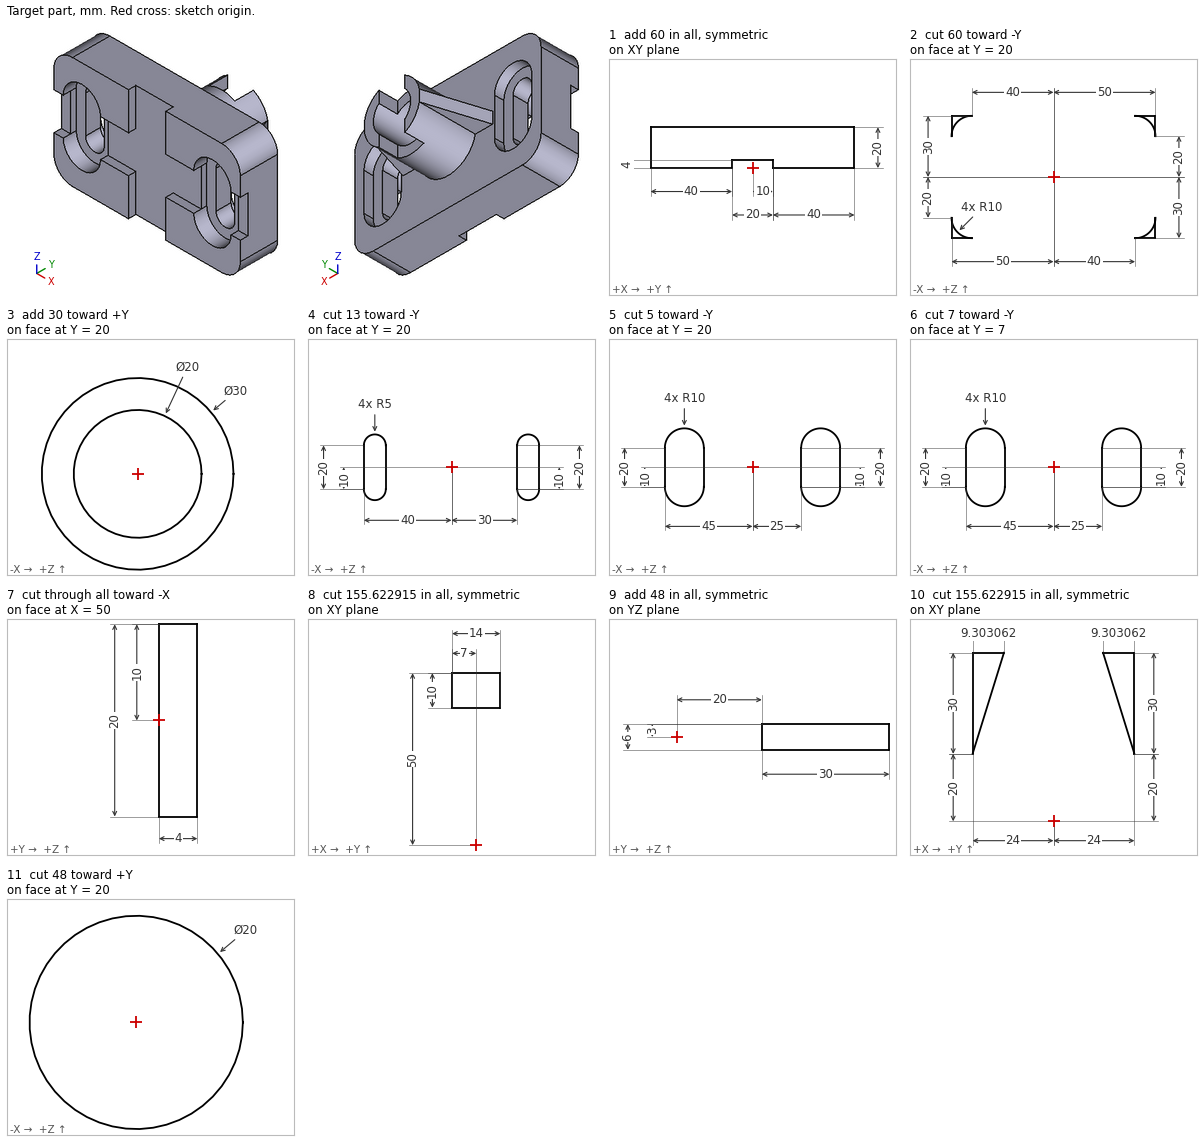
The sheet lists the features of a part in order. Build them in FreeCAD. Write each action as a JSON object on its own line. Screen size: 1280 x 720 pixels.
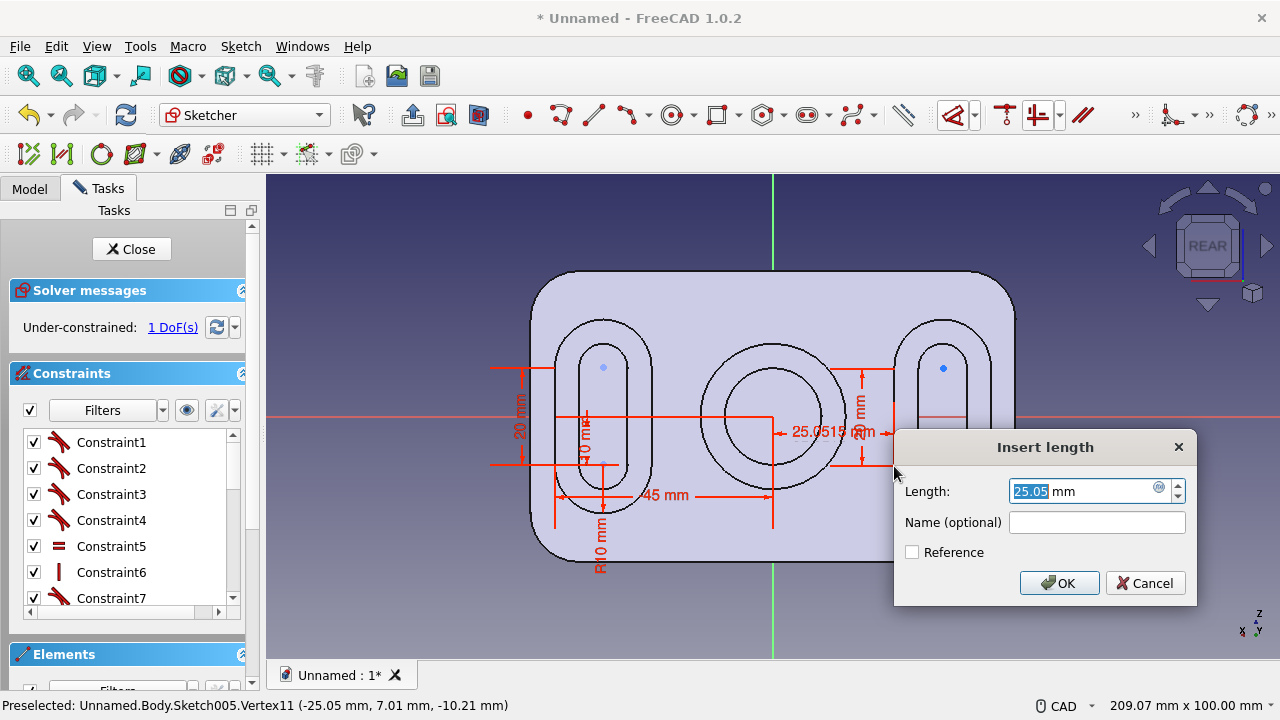
{"action": "type", "text": "25"}
{"action": "key", "text": "Return"}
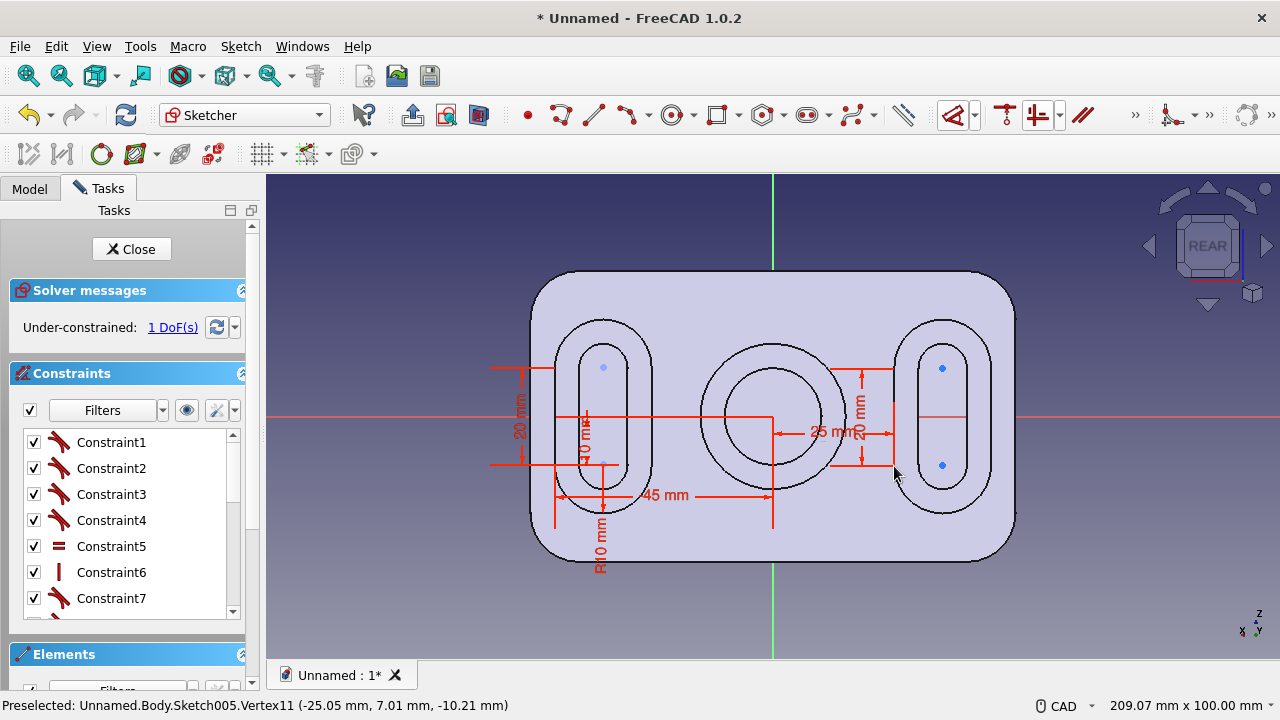
{"action": "left_click", "coordinate": [894, 466]}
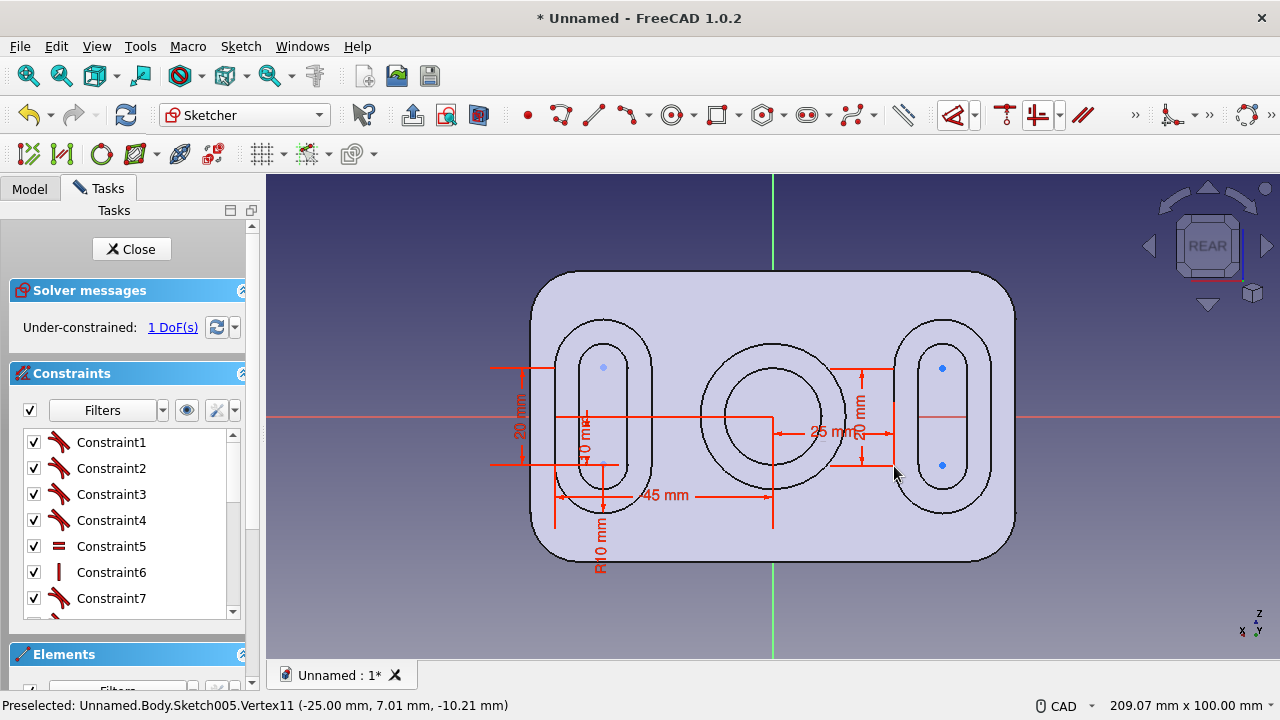
{"action": "key", "text": "i"}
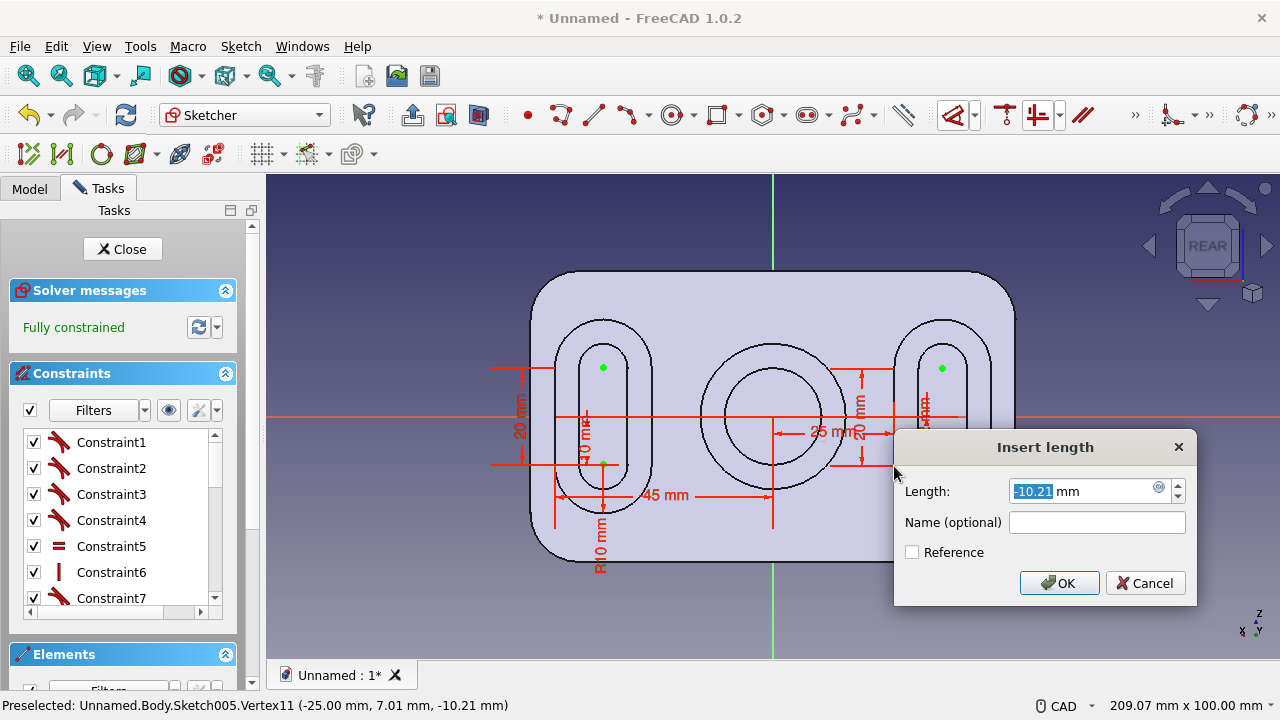
{"action": "type", "text": "-10"}
{"action": "key", "text": "Return"}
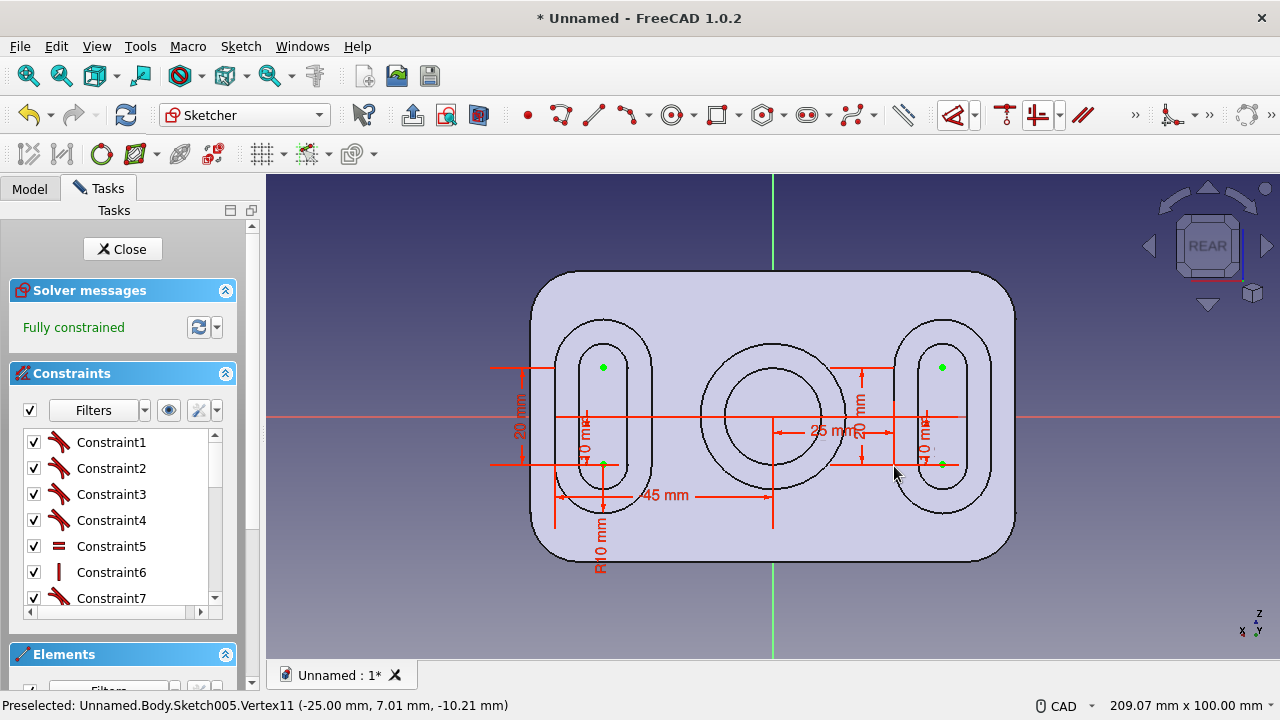
{"action": "left_click", "coordinate": [123, 249]}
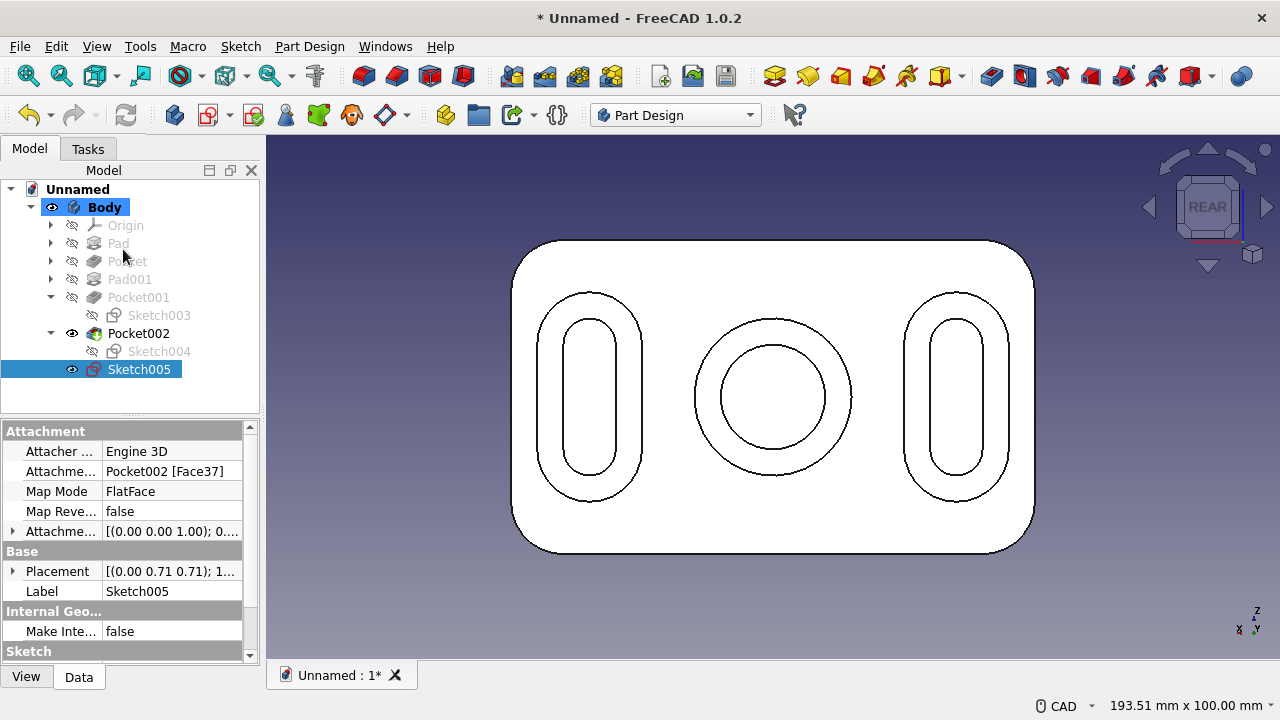
{"action": "left_click", "coordinate": [992, 76]}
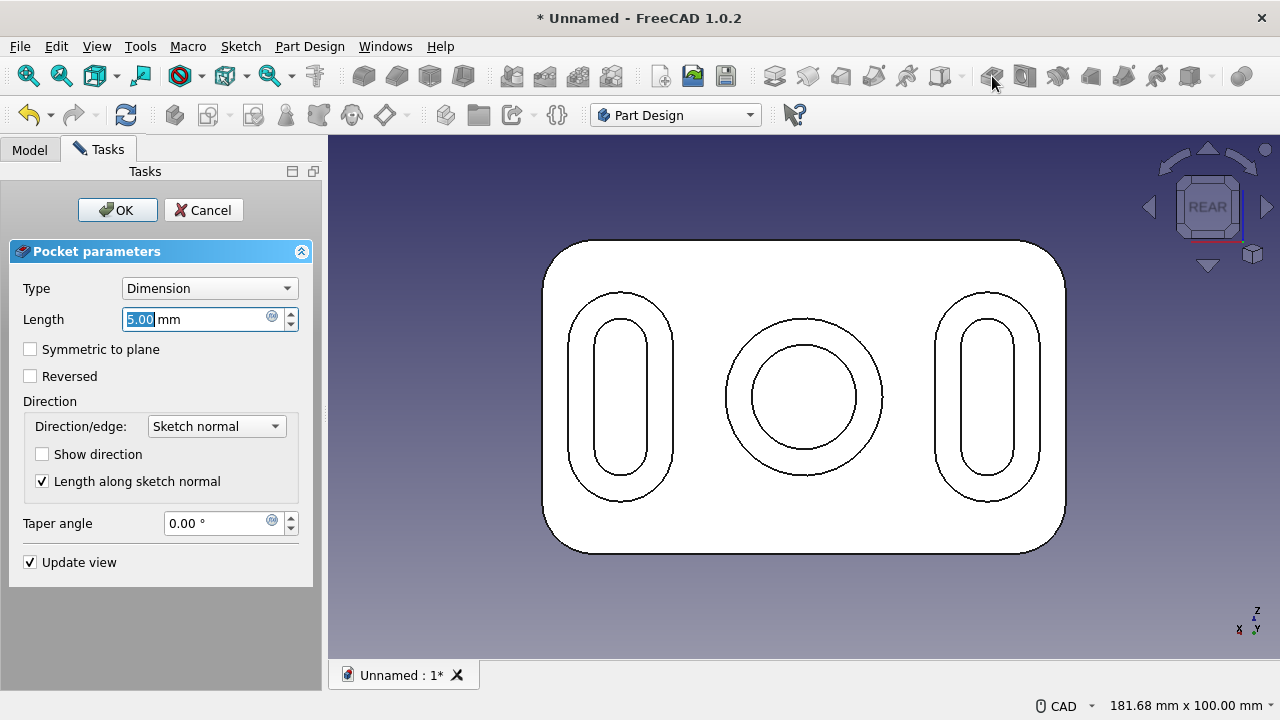
{"action": "type", "text": "7"}
{"action": "key", "text": "Tab"}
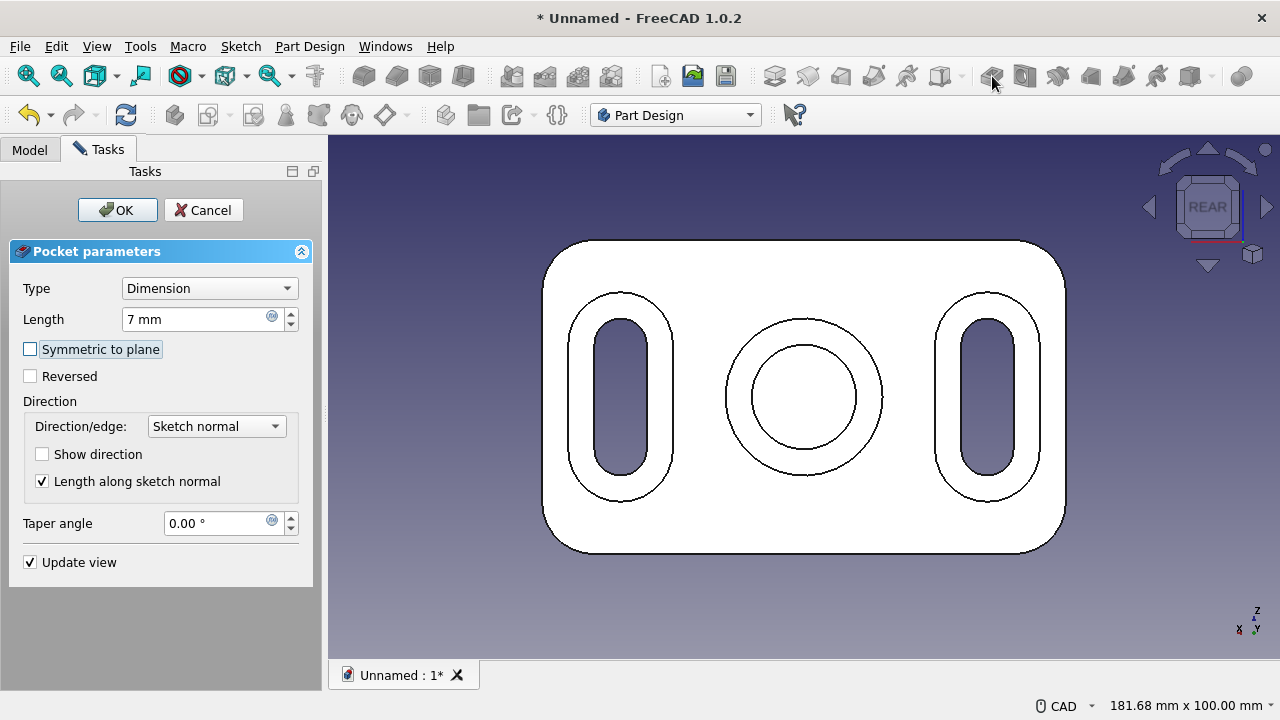
{"action": "left_click", "coordinate": [118, 210]}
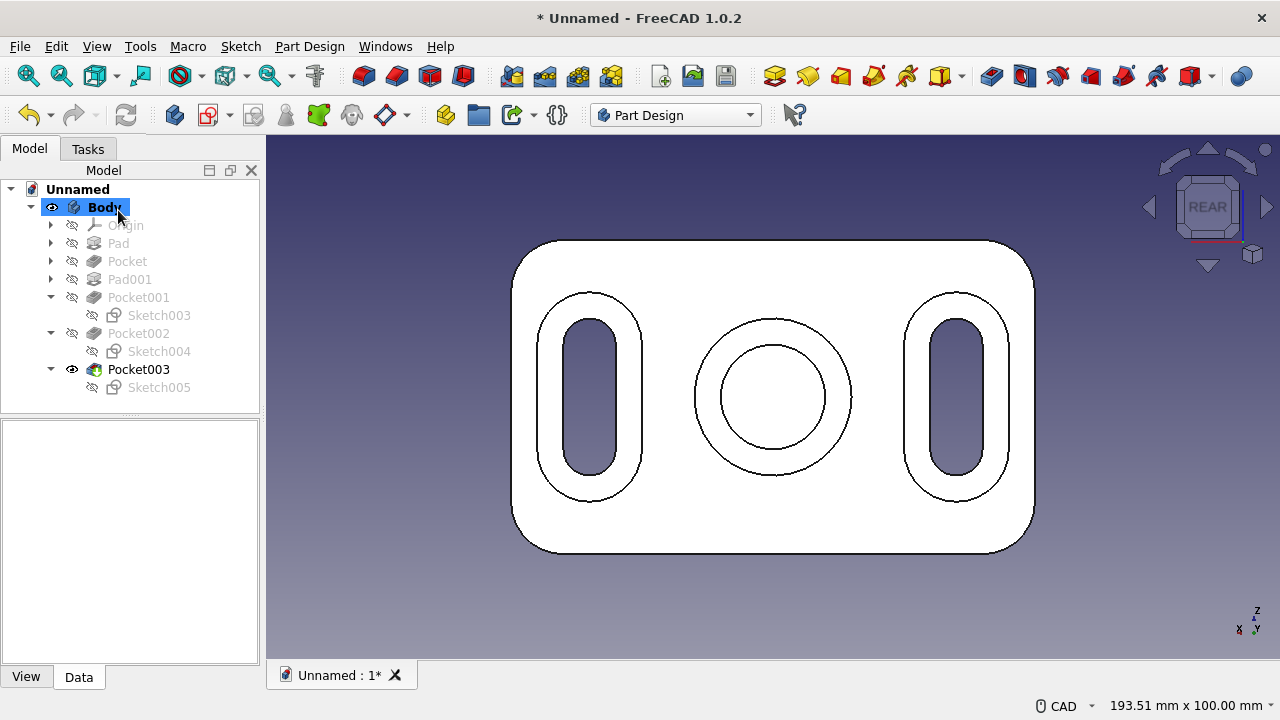
{"action": "key", "text": "0"}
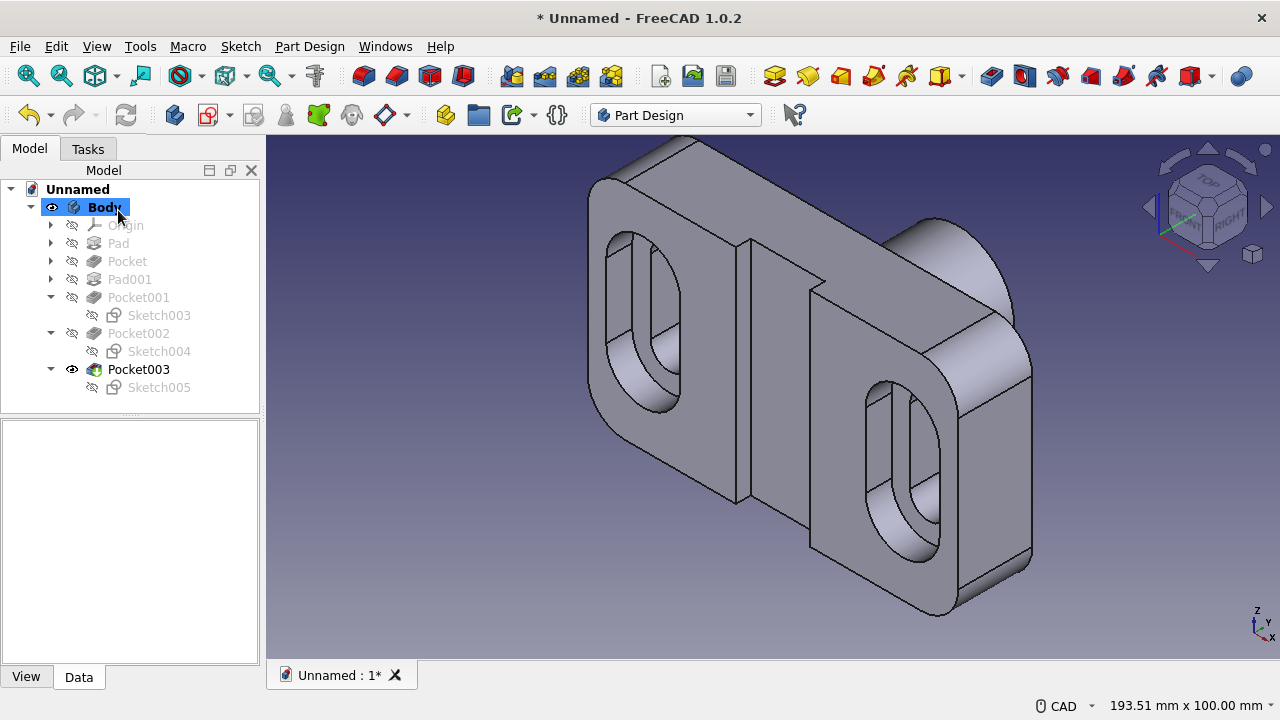
{"action": "key", "text": "v f"}